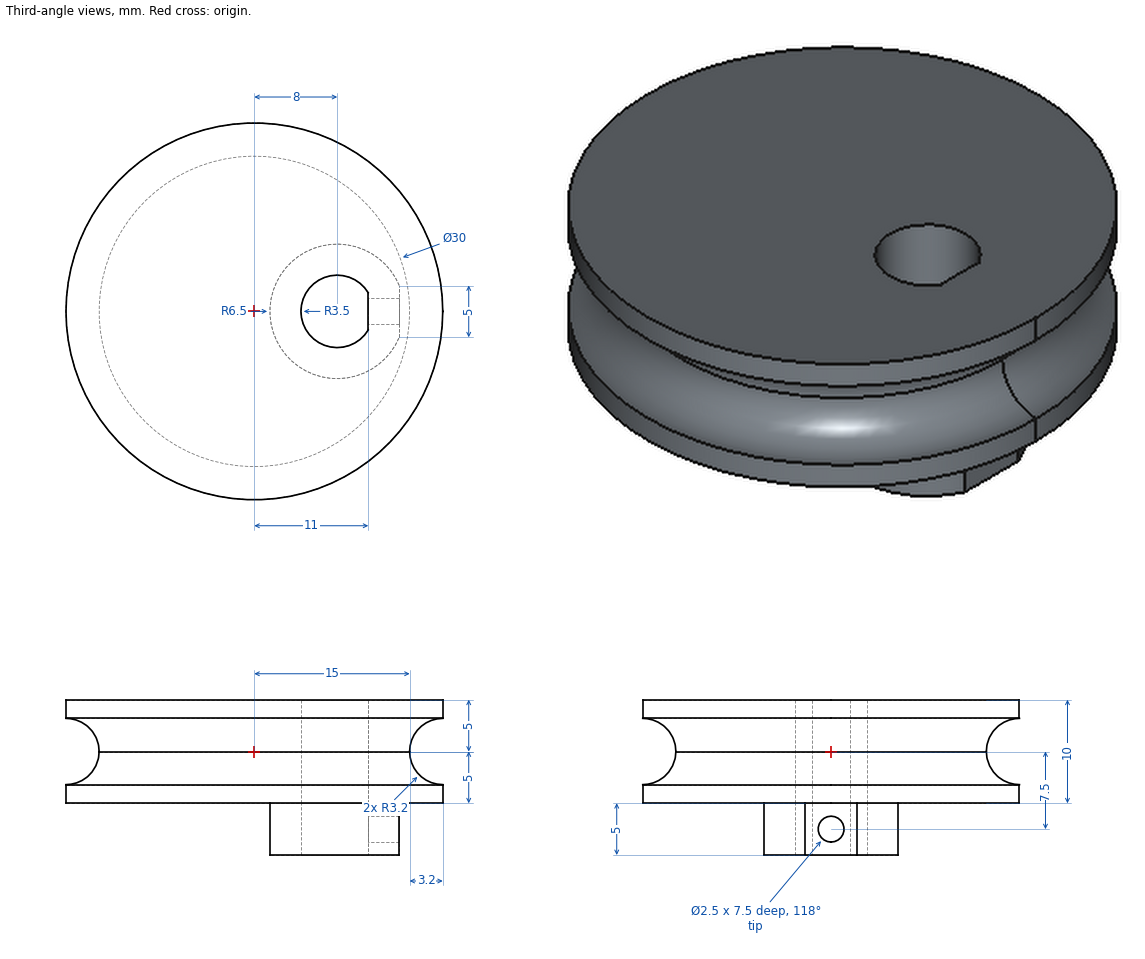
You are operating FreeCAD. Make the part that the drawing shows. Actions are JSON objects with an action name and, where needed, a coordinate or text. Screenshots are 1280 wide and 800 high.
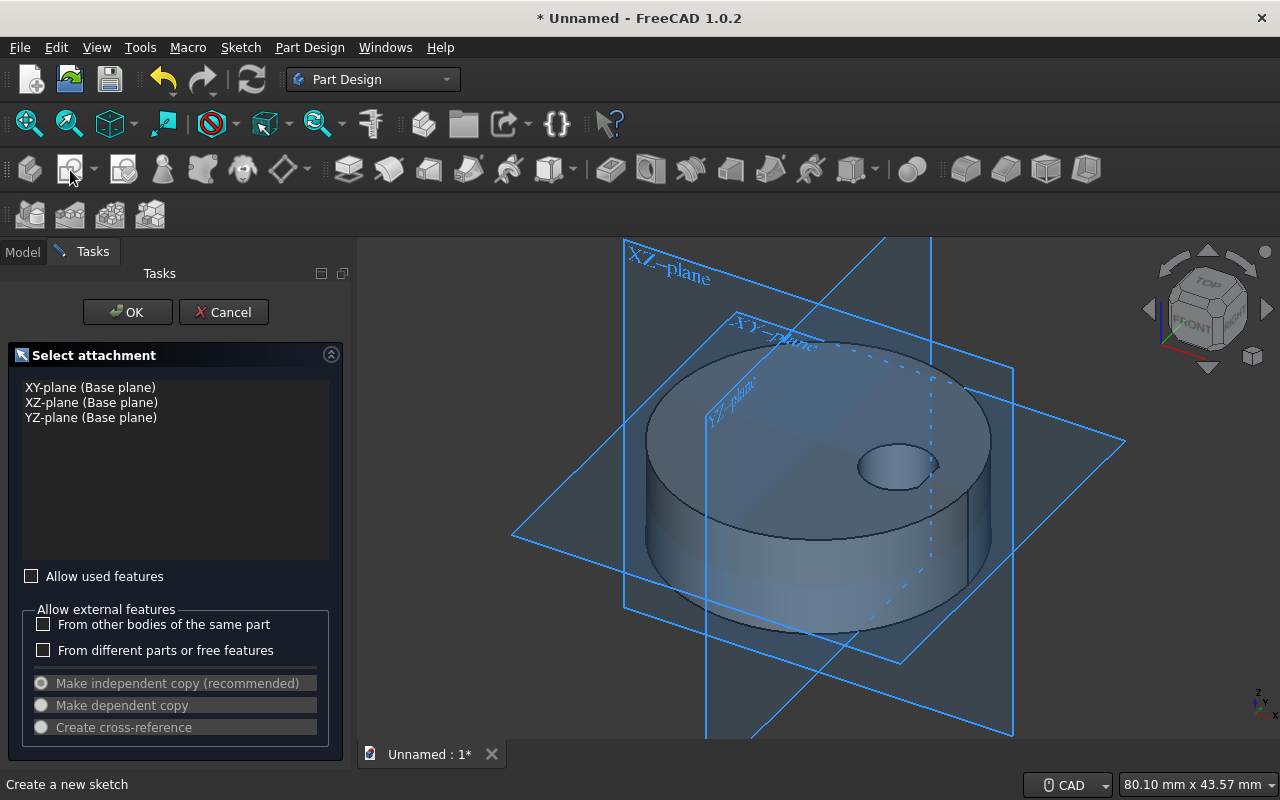
{"action": "left_click", "coordinate": [82, 402]}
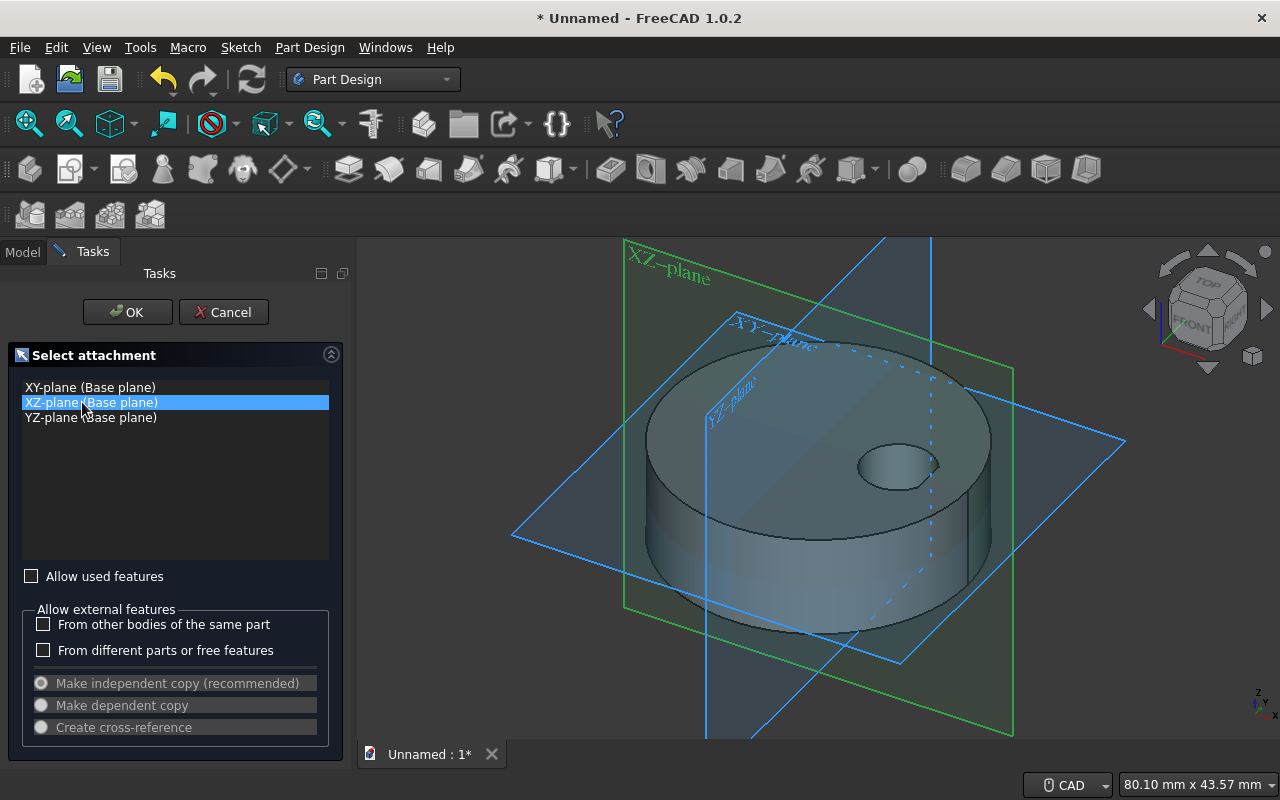
{"action": "left_click", "coordinate": [128, 312]}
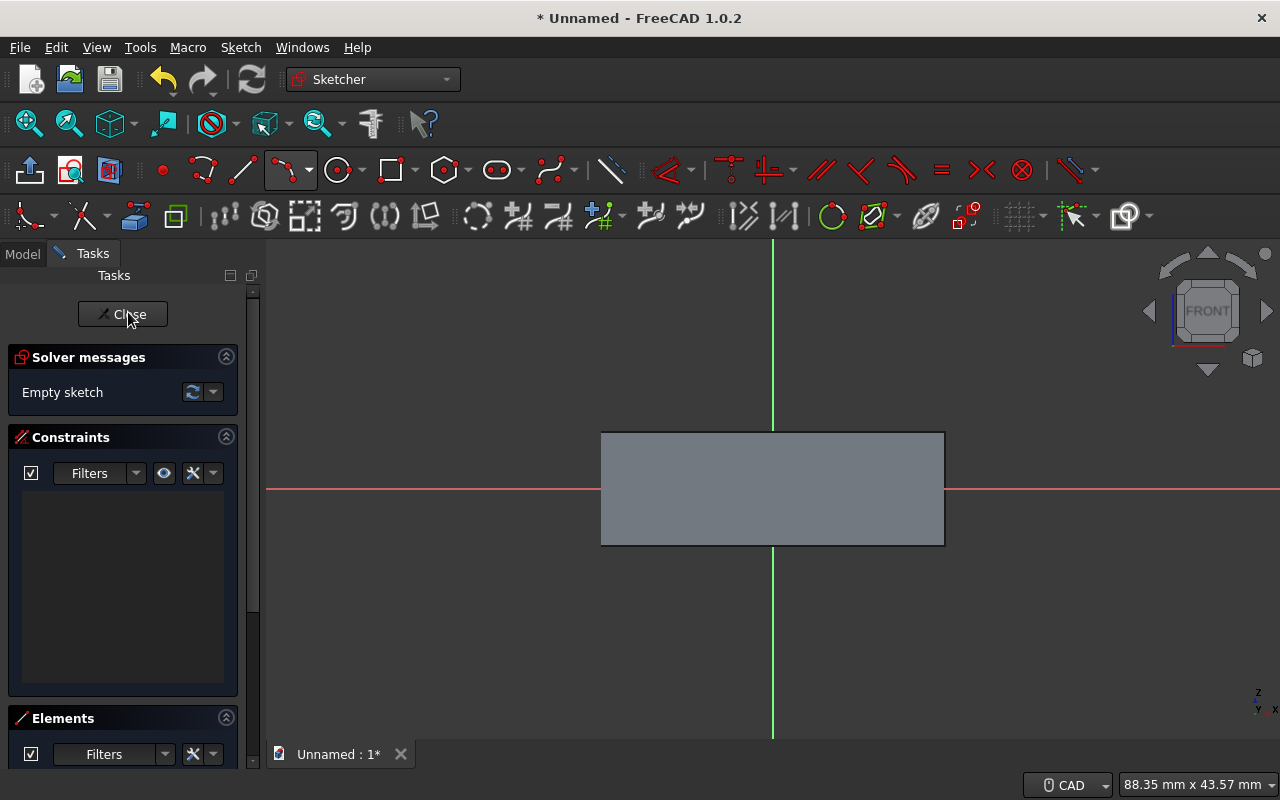
{"action": "left_click", "coordinate": [110, 170]}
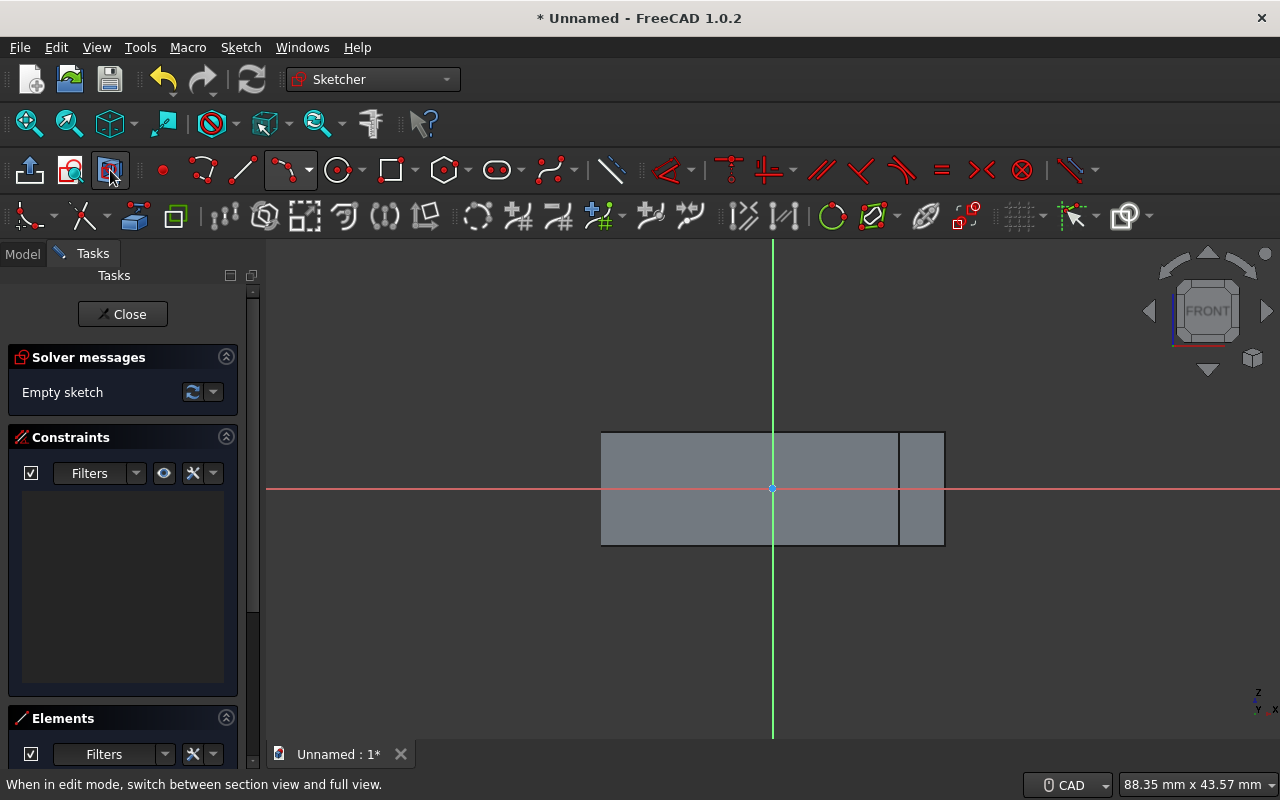
{"action": "scroll", "coordinate": [978, 489], "scroll_direction": "up", "scroll_amount": 5}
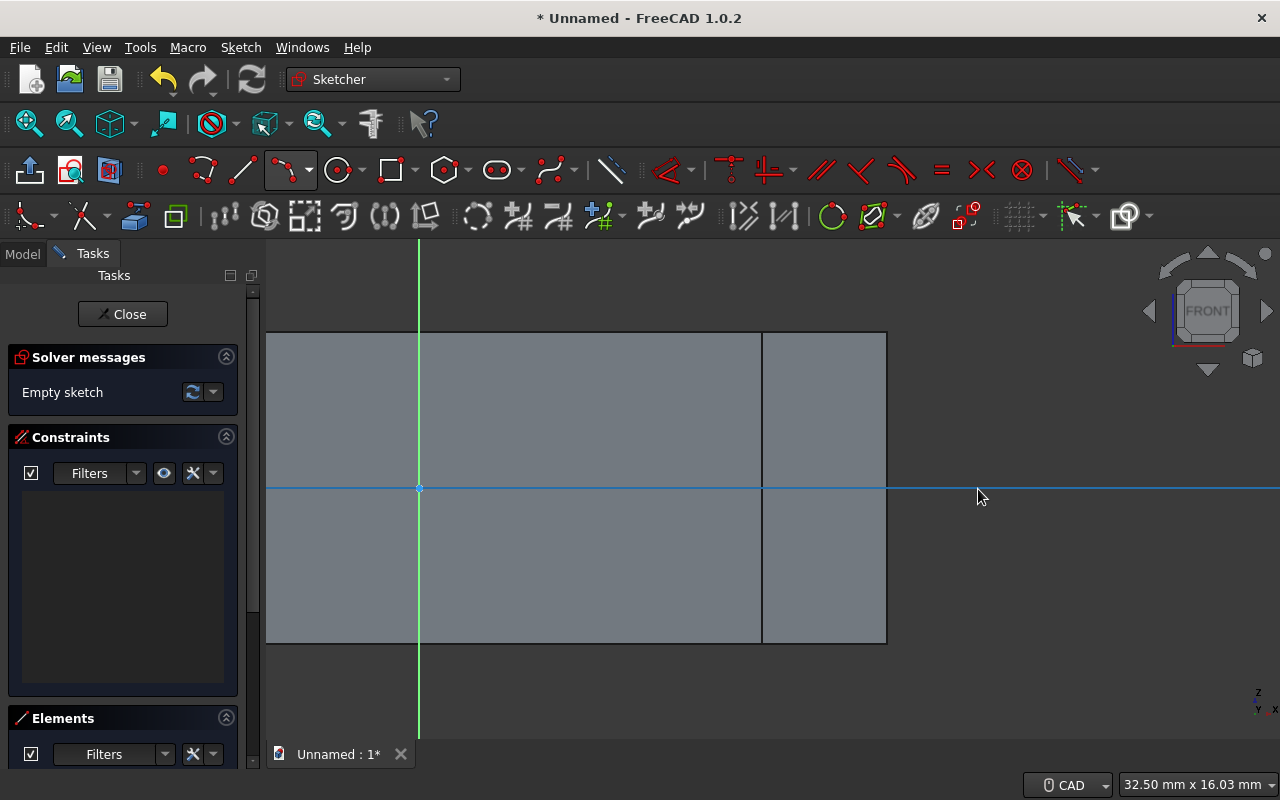
{"action": "left_click", "coordinate": [204, 170]}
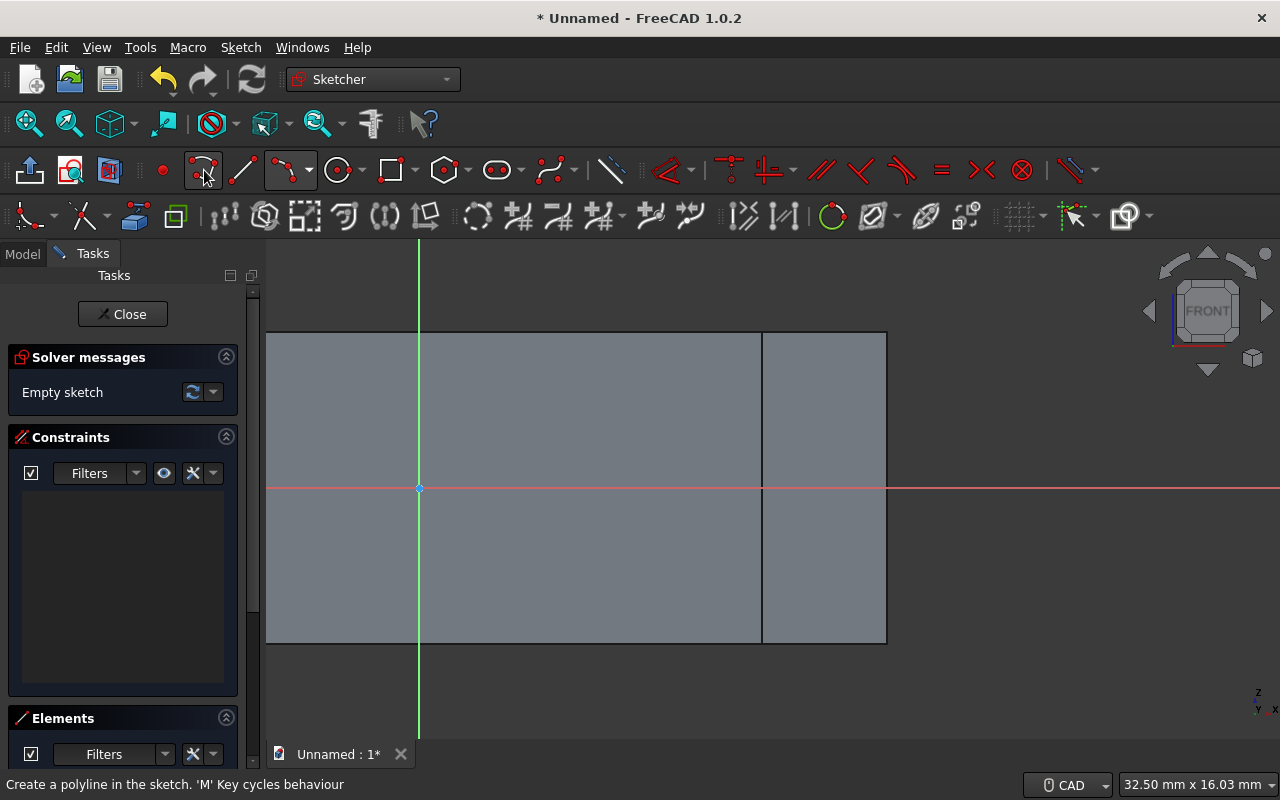
{"action": "left_click", "coordinate": [987, 588]}
{"action": "left_click", "coordinate": [987, 644]}
{"action": "left_click", "coordinate": [887, 644]}
{"action": "left_click", "coordinate": [887, 488]}
{"action": "right_click", "coordinate": [887, 488]}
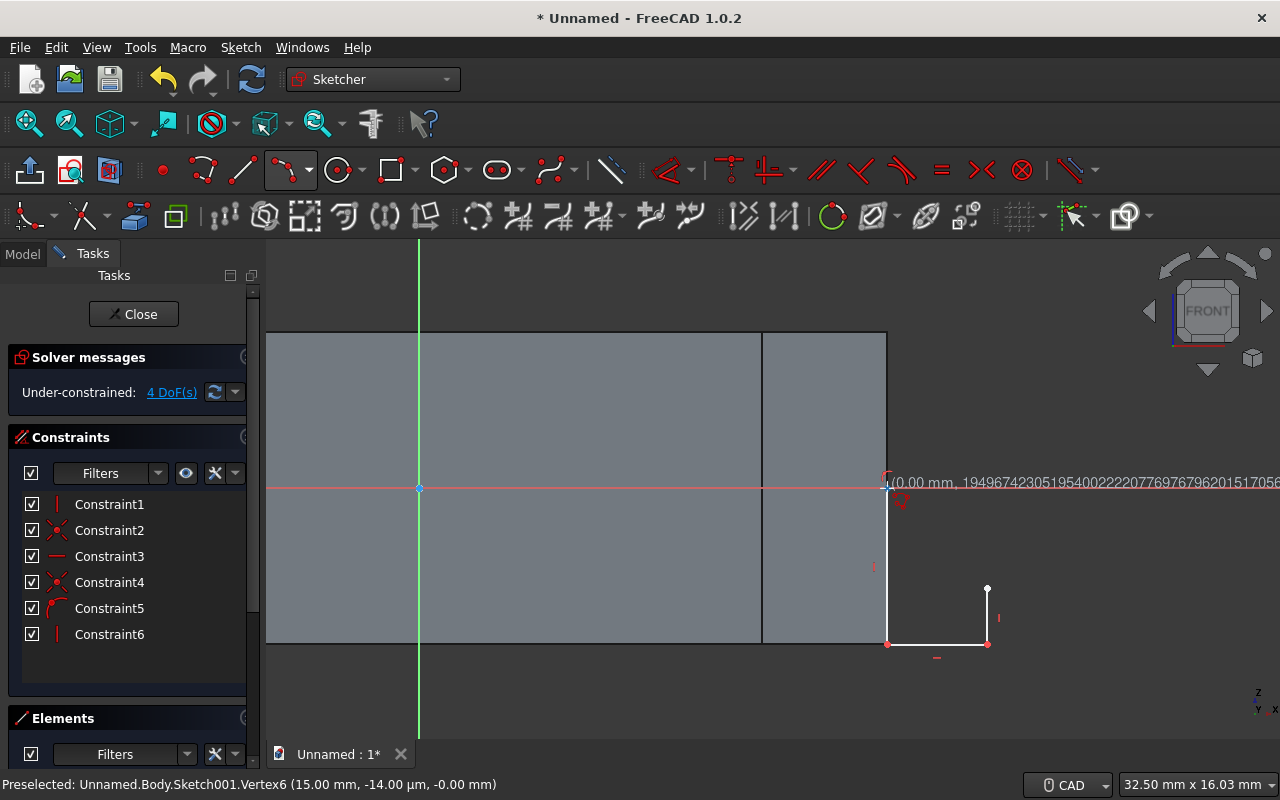
{"action": "left_click", "coordinate": [284, 170]}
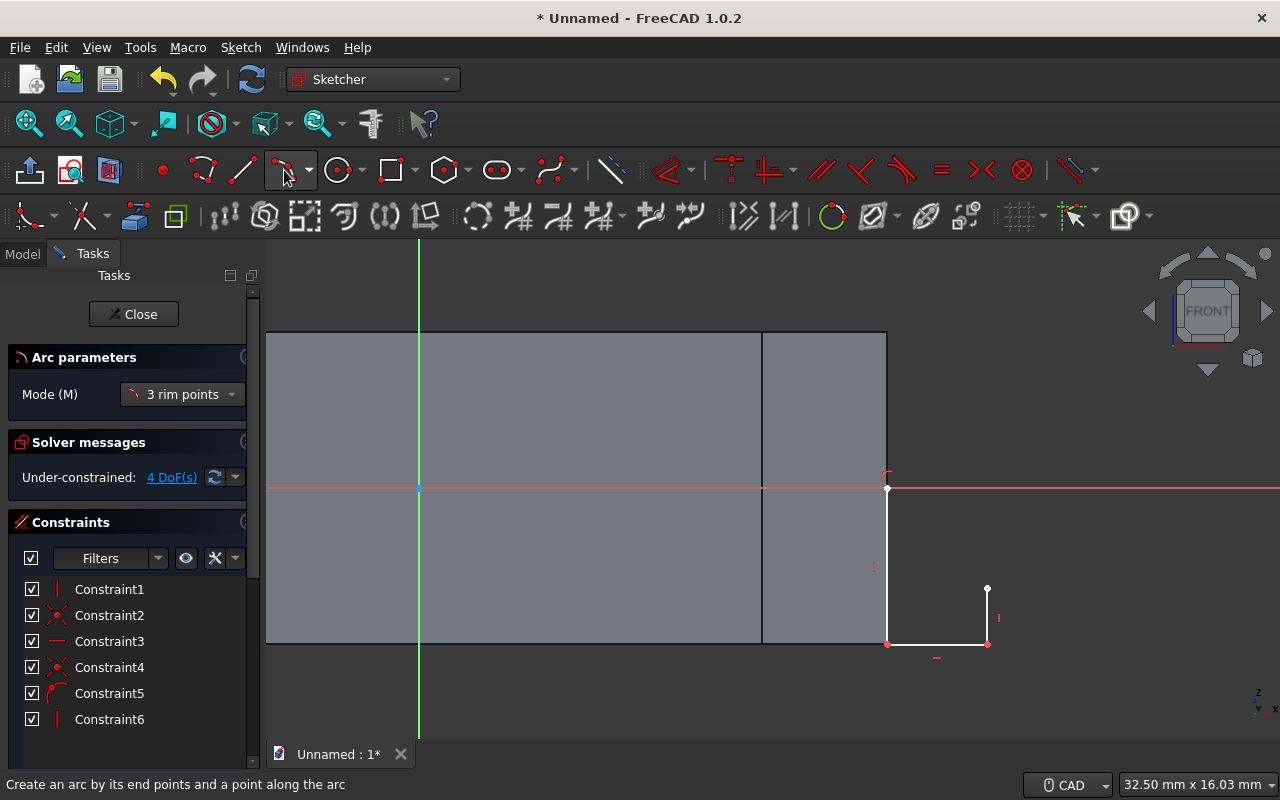
{"action": "left_click", "coordinate": [887, 488]}
{"action": "left_click", "coordinate": [987, 589]}
{"action": "left_click", "coordinate": [916, 559]}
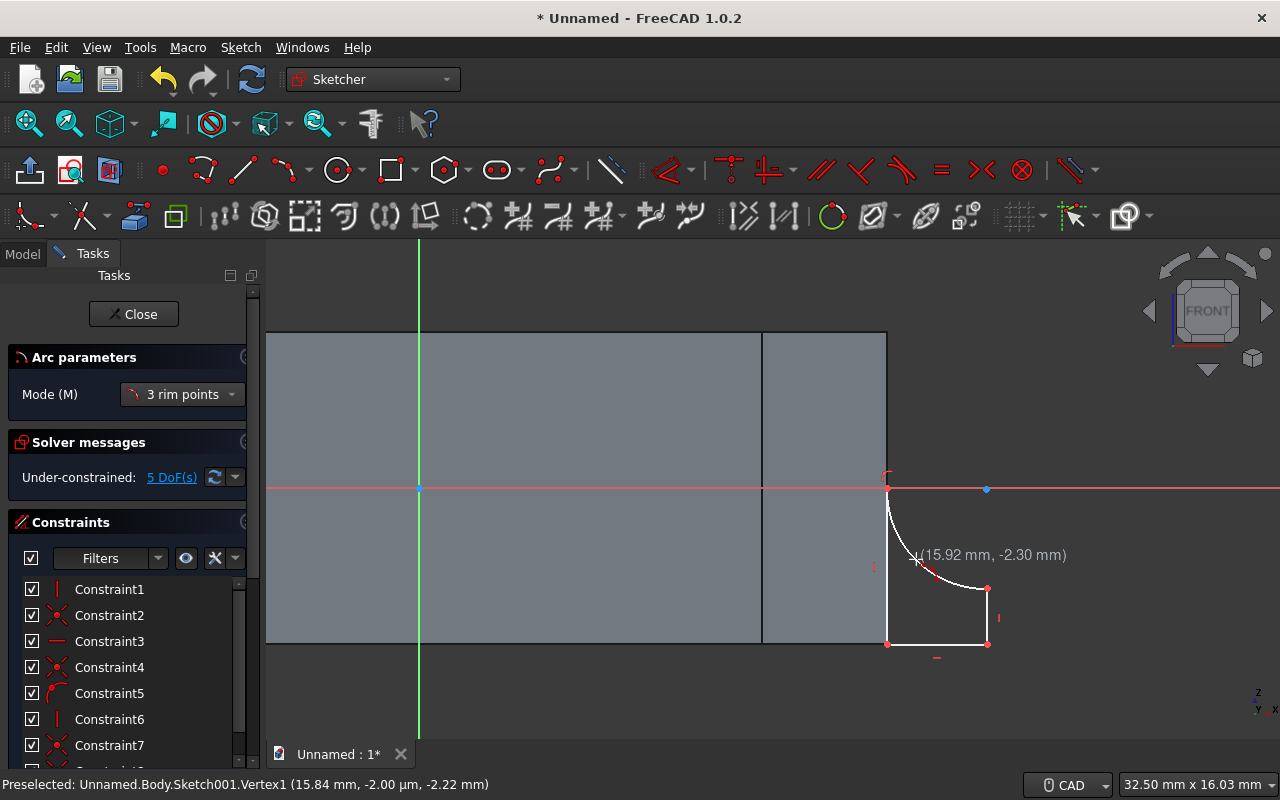
{"action": "left_click", "coordinate": [204, 170]}